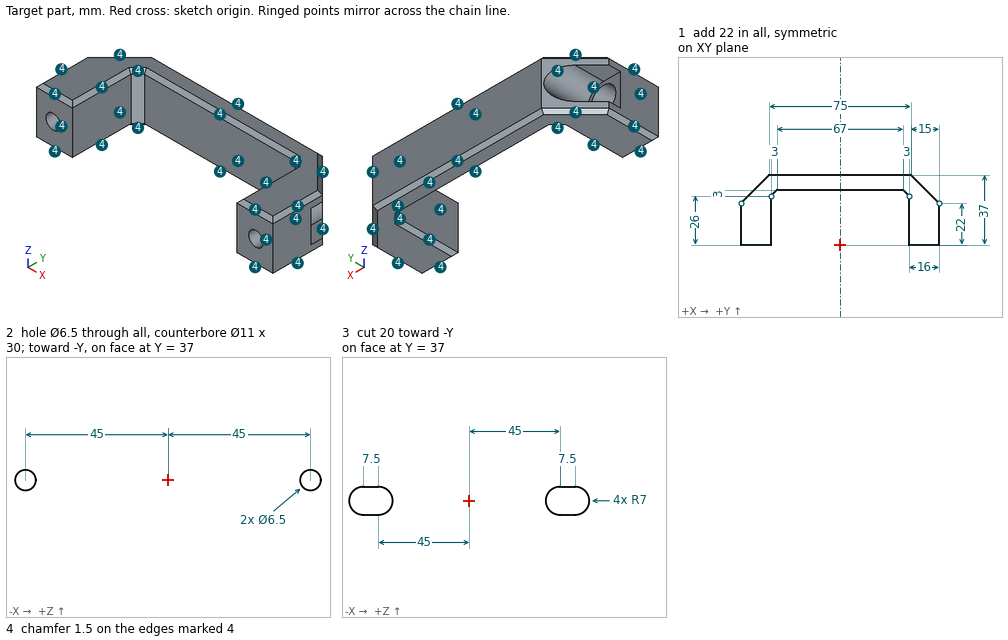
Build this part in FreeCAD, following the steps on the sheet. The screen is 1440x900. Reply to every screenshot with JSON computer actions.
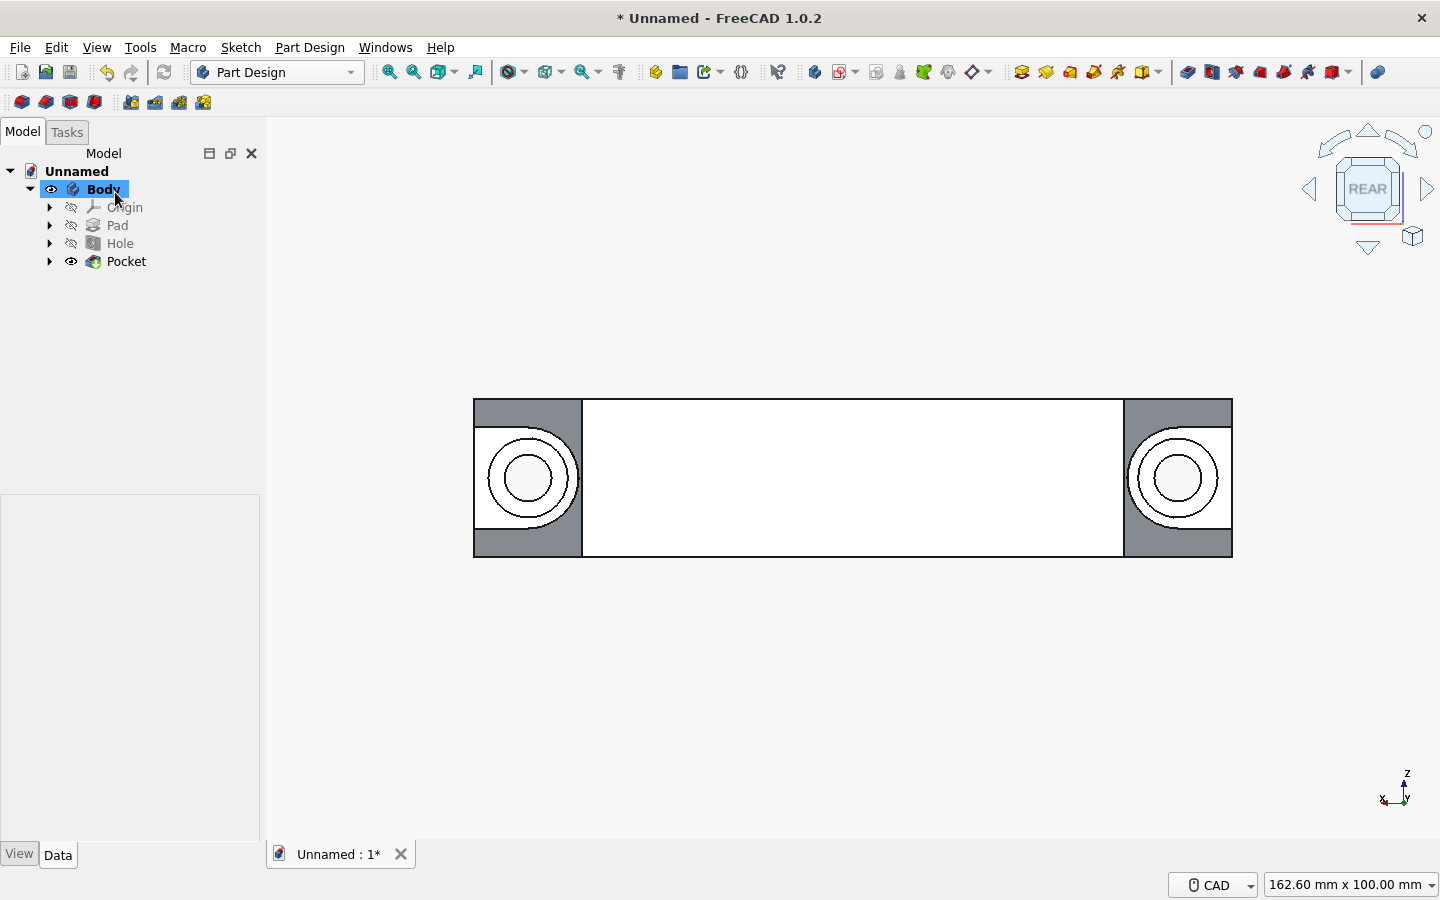
{"action": "key", "text": "0"}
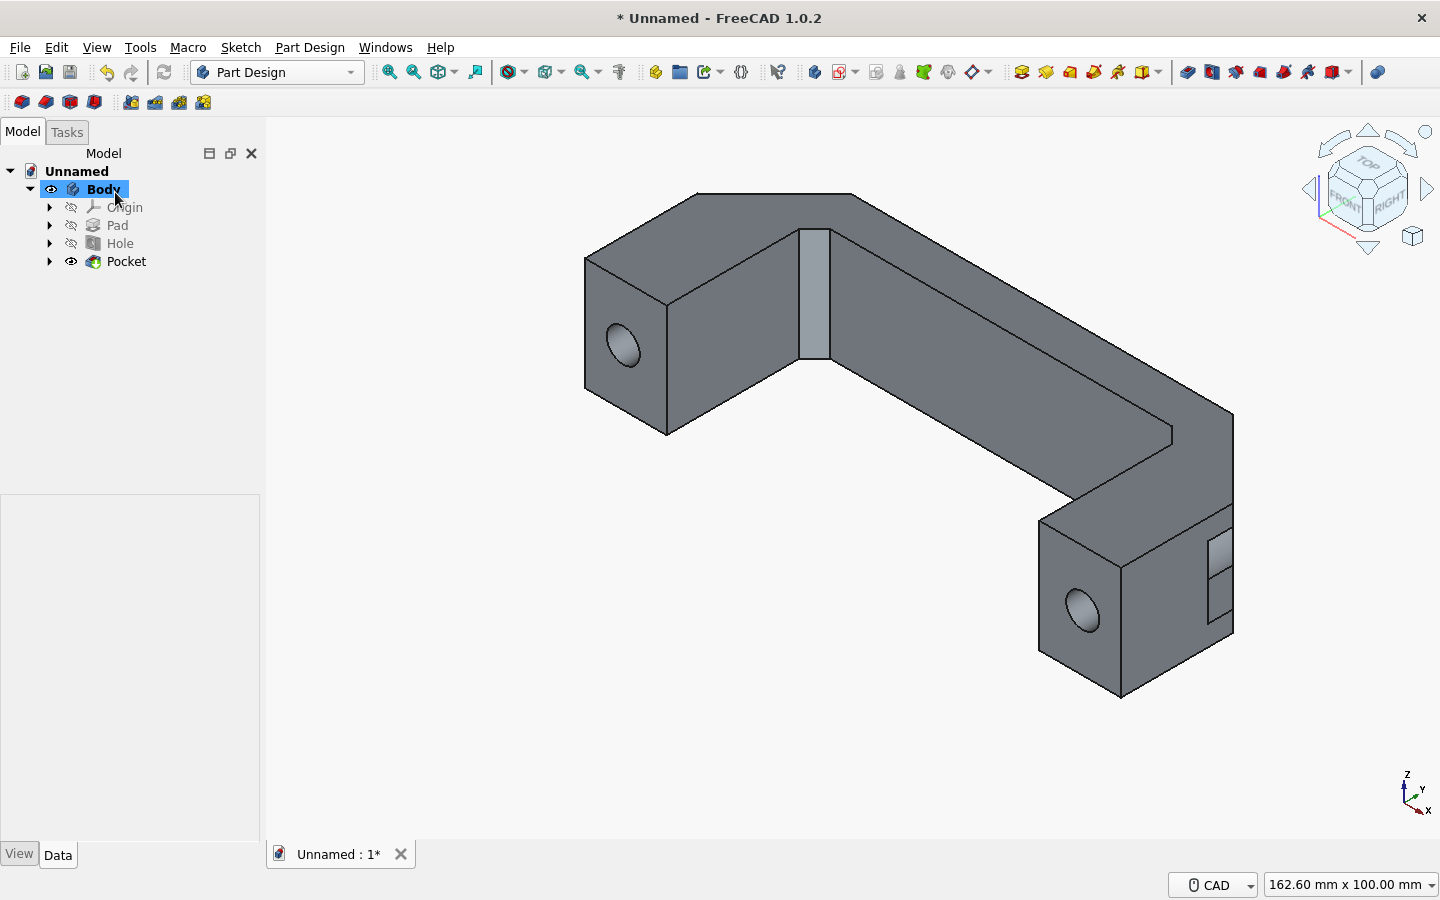
{"action": "left_click", "coordinate": [1177, 490]}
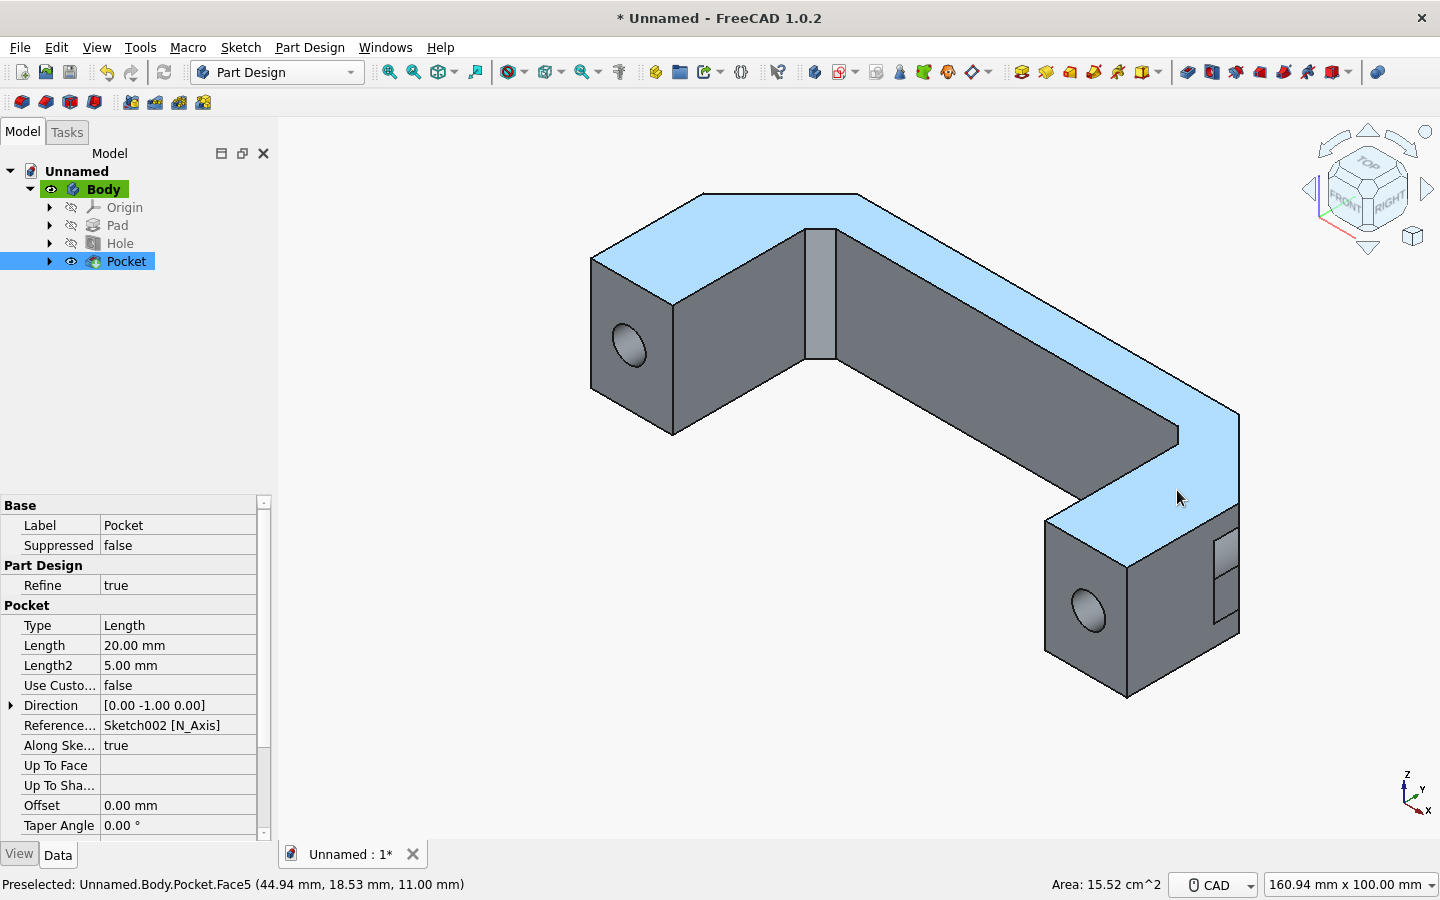
{"action": "key", "text": "2"}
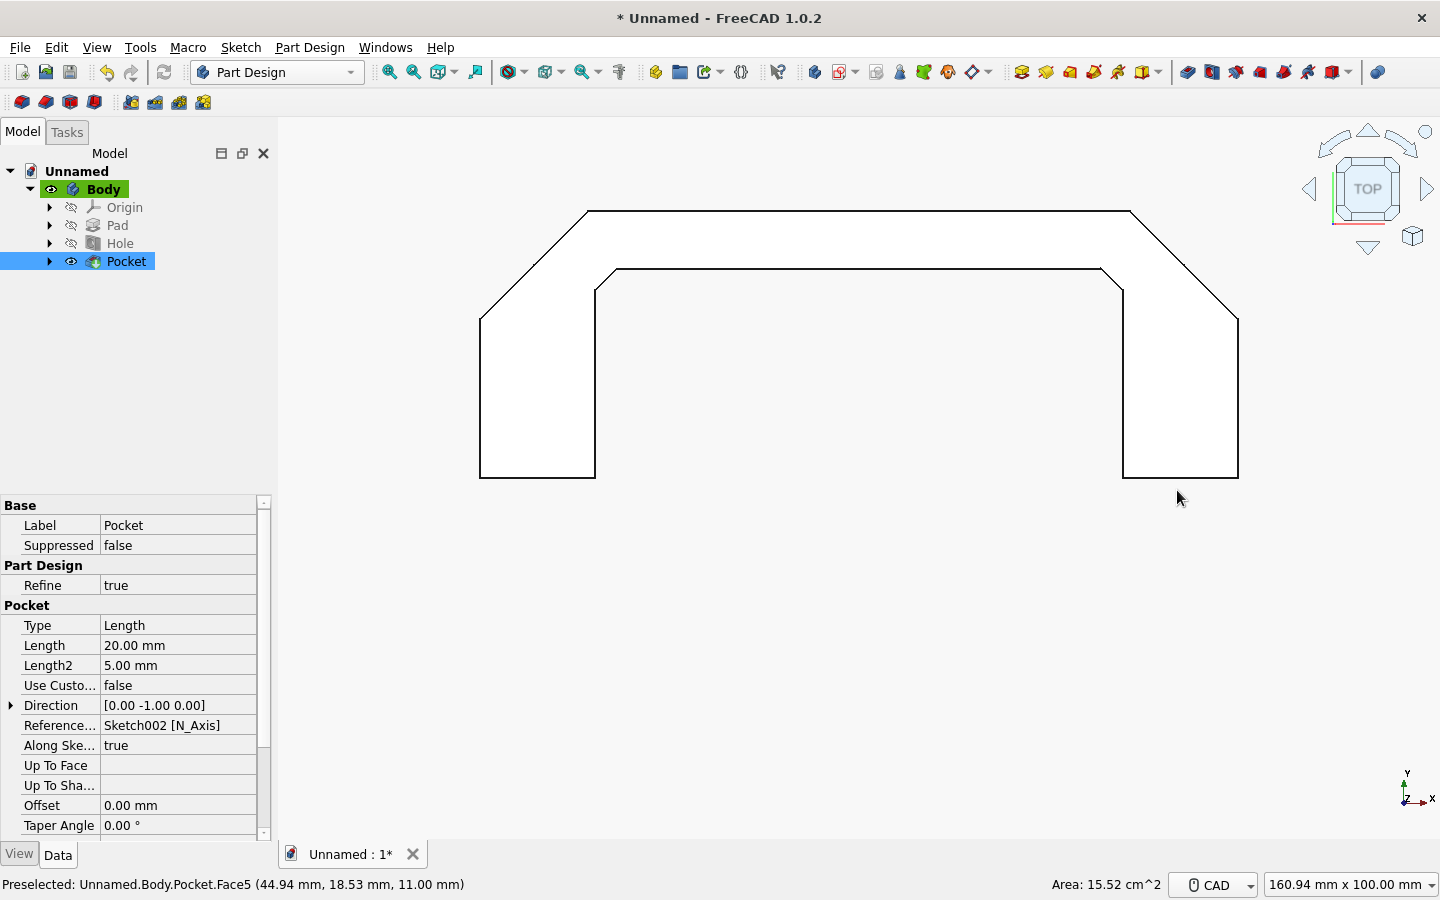
{"action": "key", "text": "1"}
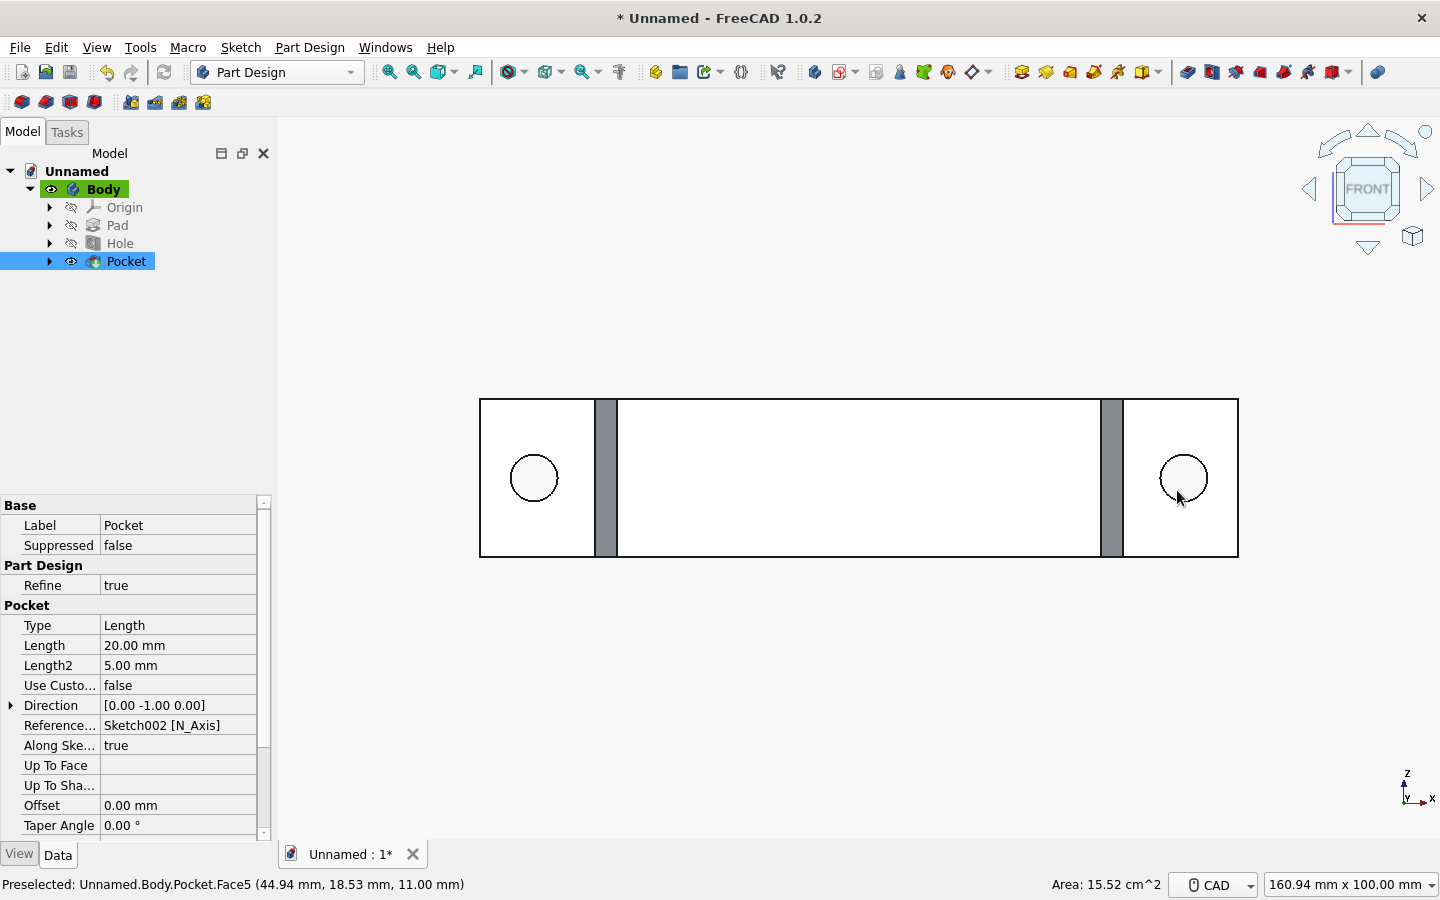
{"action": "key", "text": "3"}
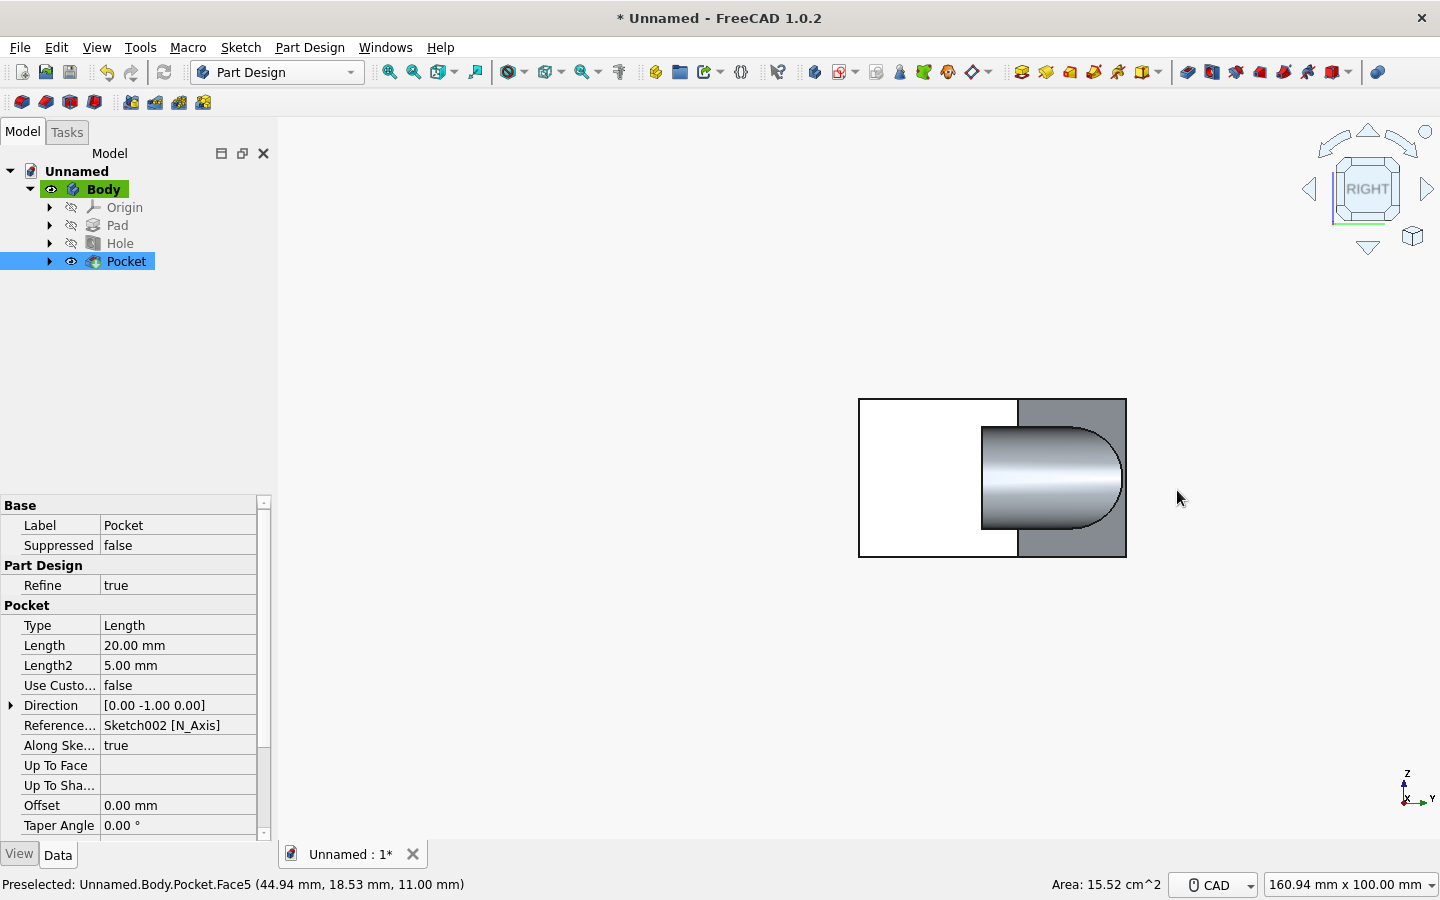
{"action": "left_click", "coordinate": [390, 72]}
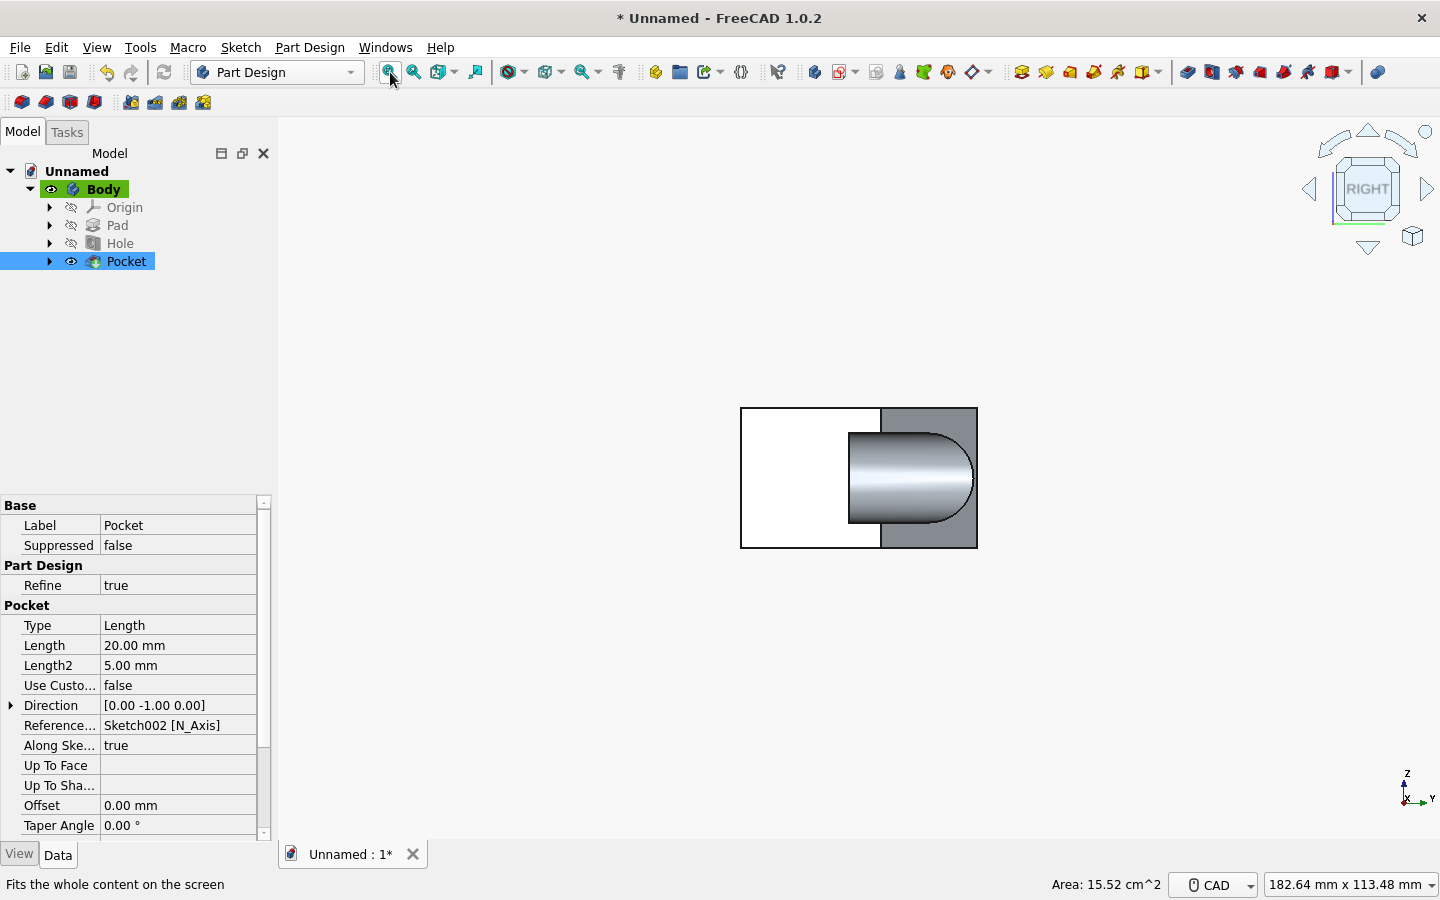
{"action": "key", "text": "5"}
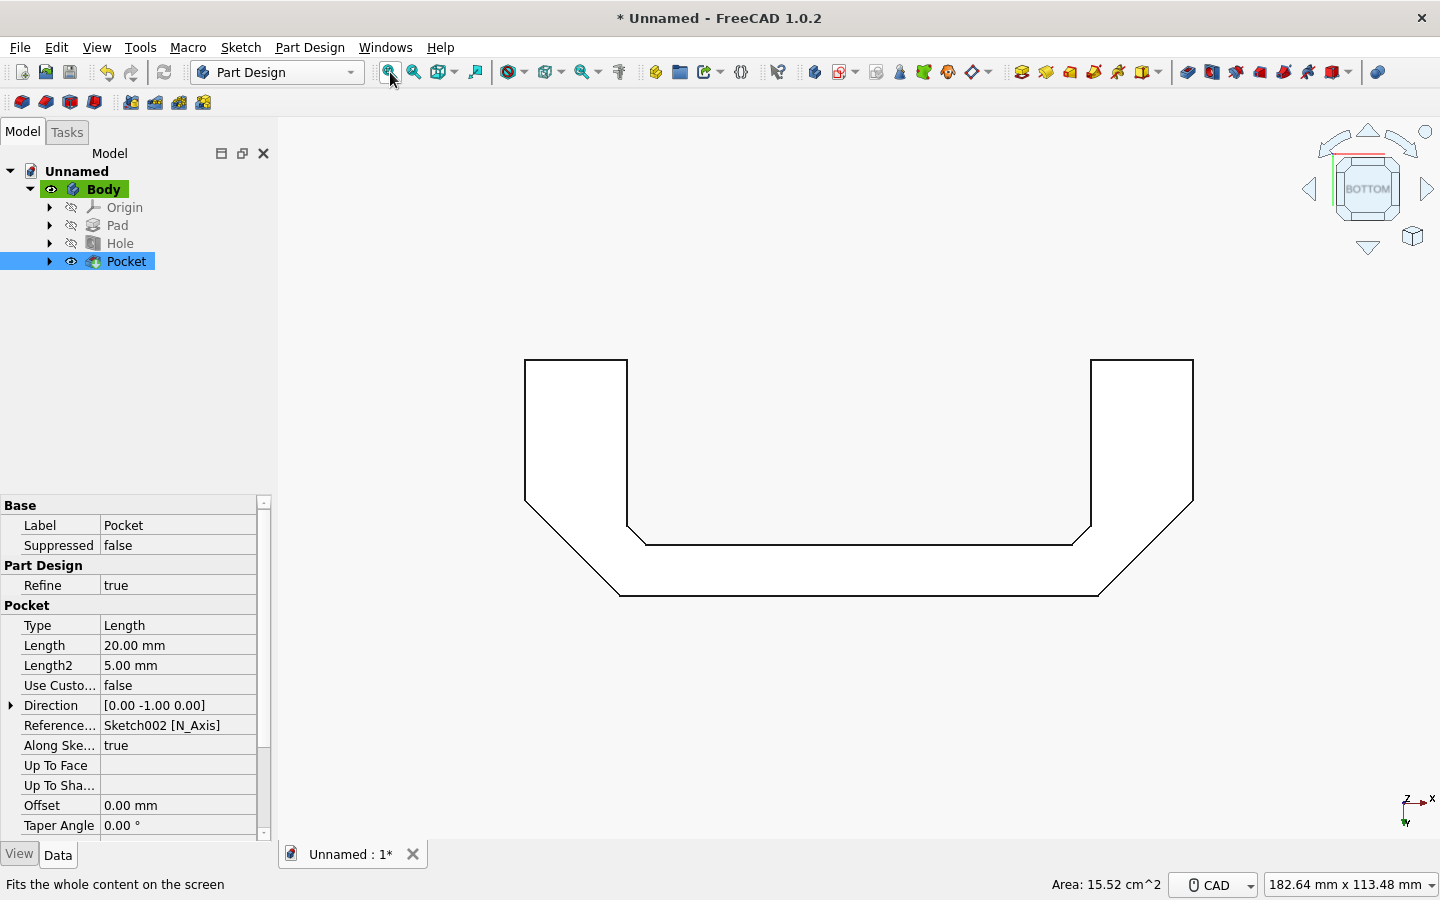
{"action": "left_click", "coordinate": [1145, 477], "text": "ctrl"}